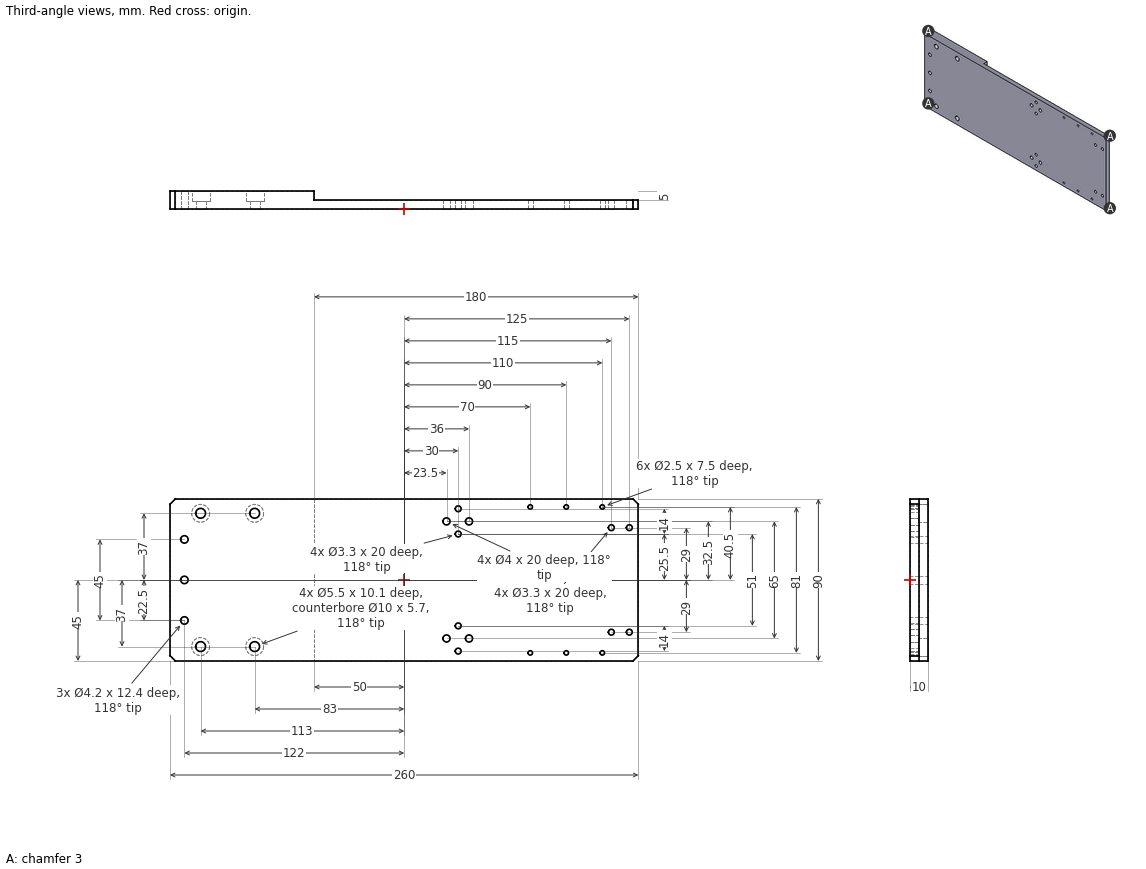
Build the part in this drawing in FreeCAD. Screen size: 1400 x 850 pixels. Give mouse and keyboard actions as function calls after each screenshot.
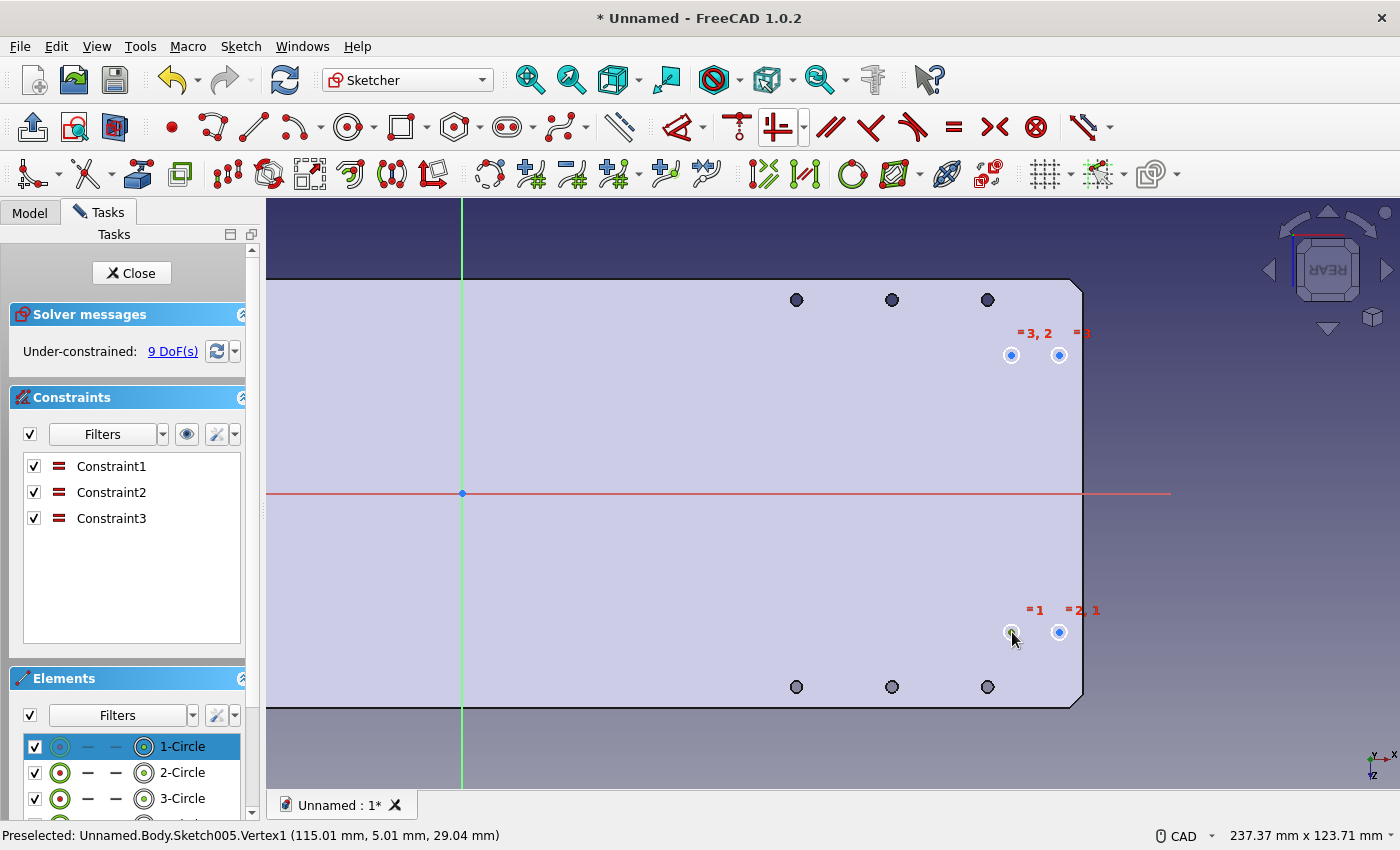
click(1059, 632)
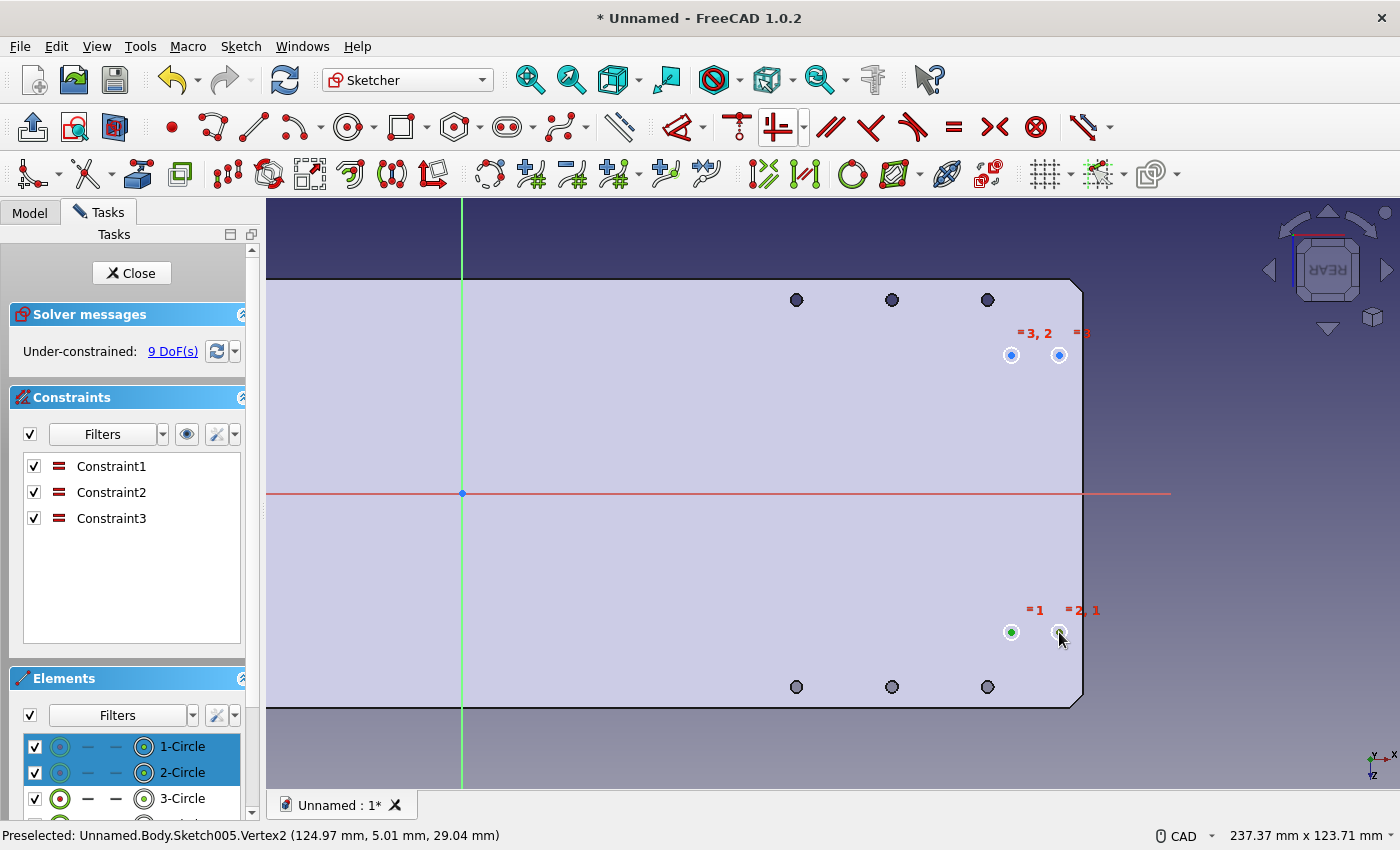
click(804, 128)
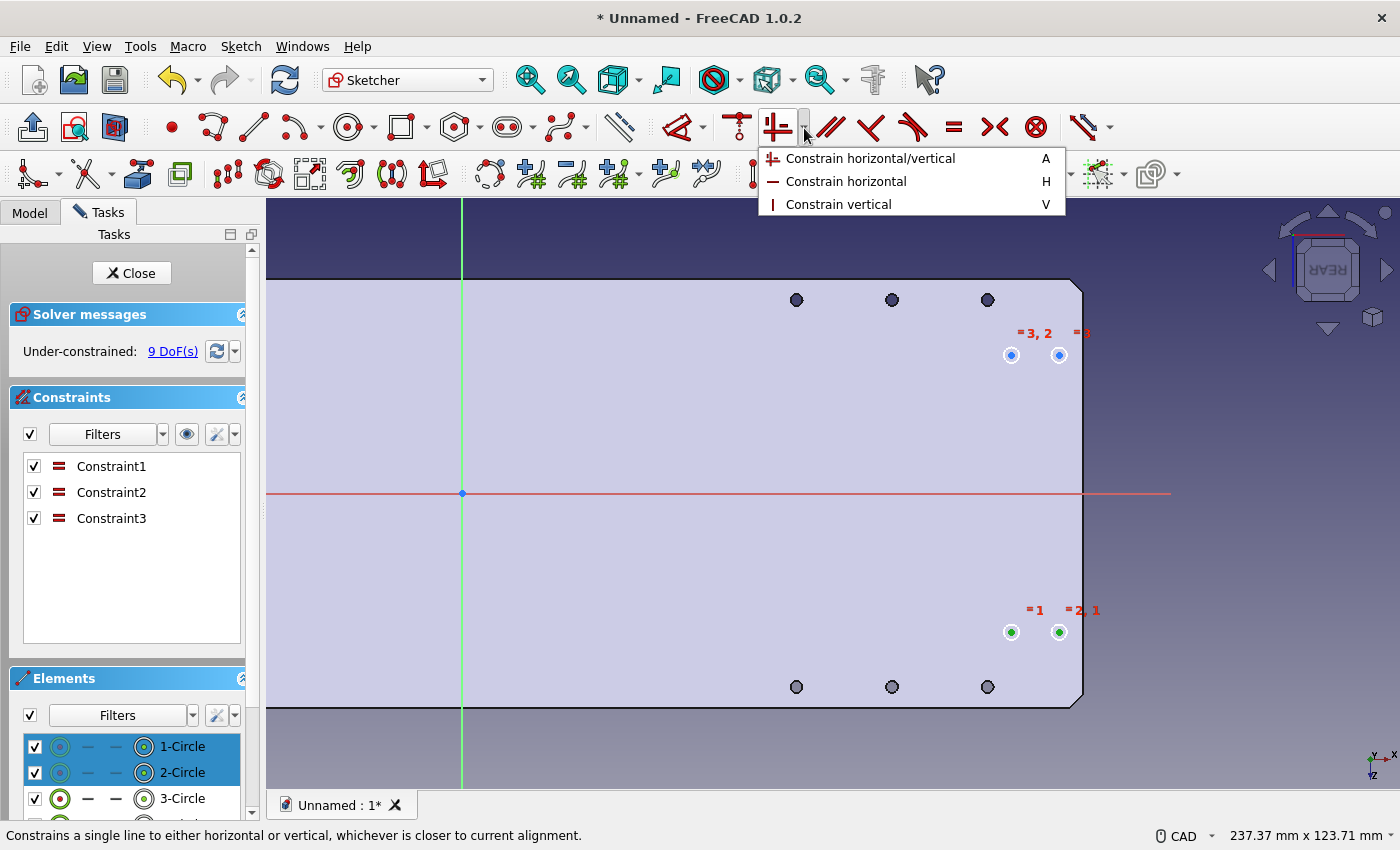
click(912, 182)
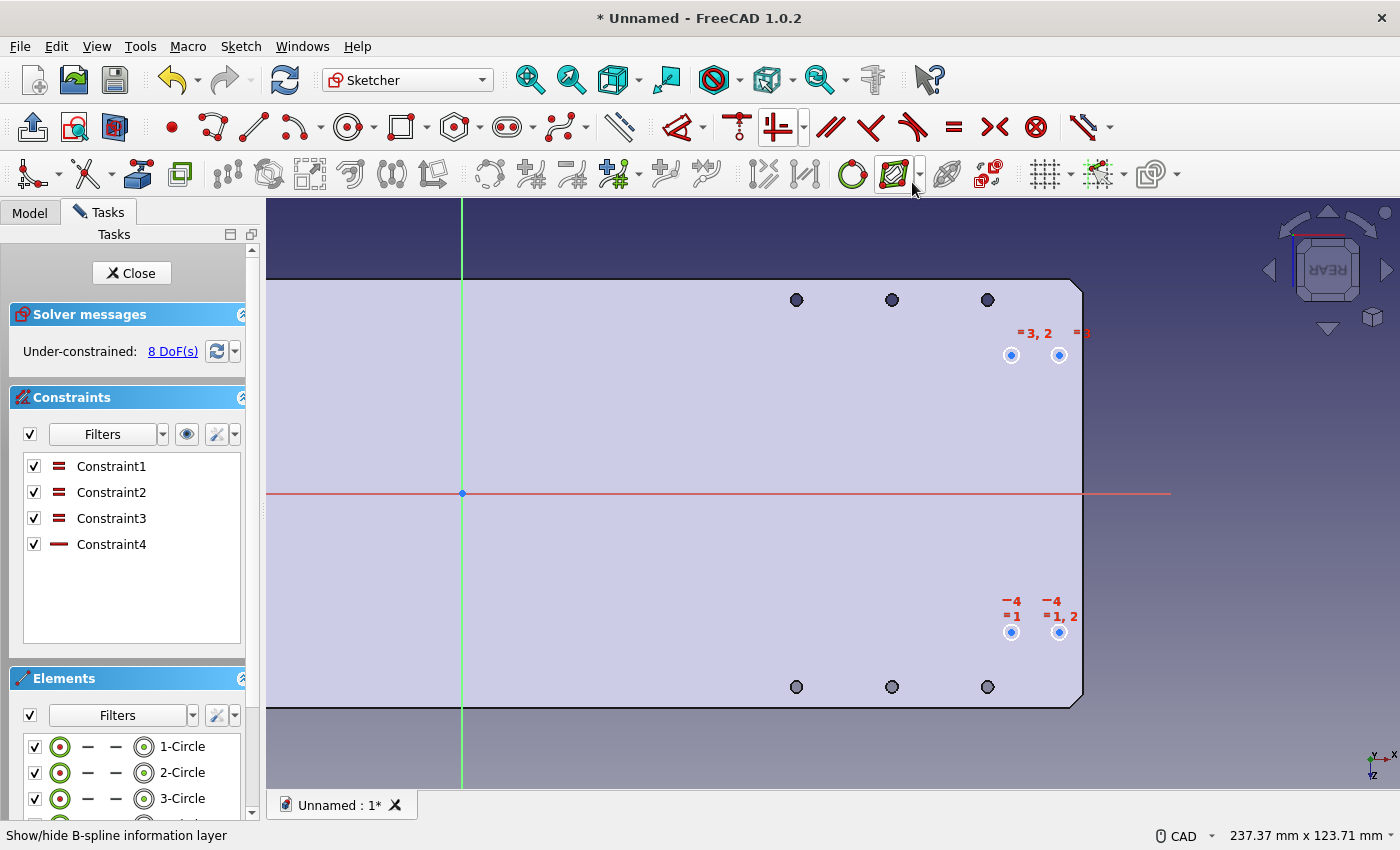
click(1012, 632)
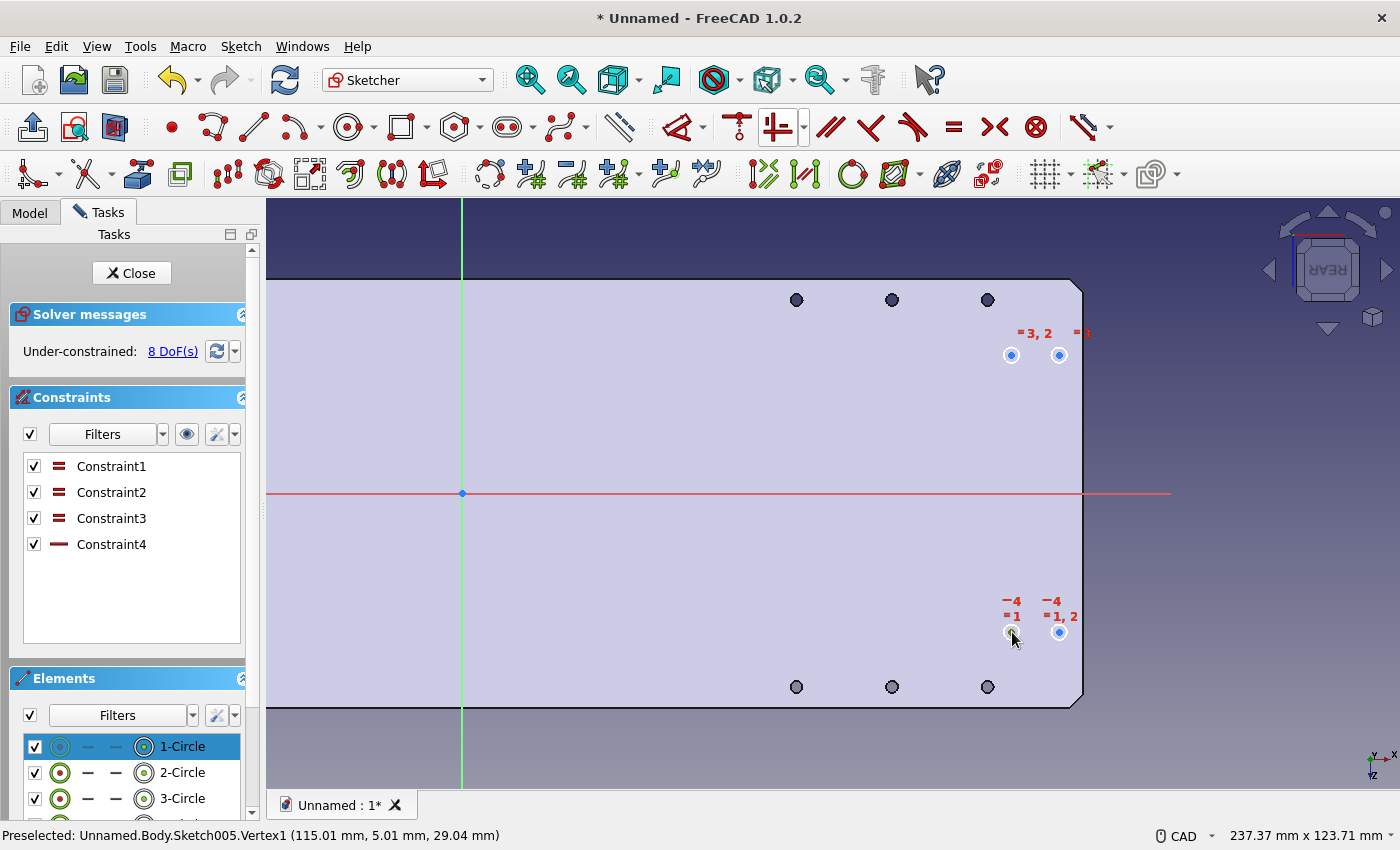
click(1012, 355)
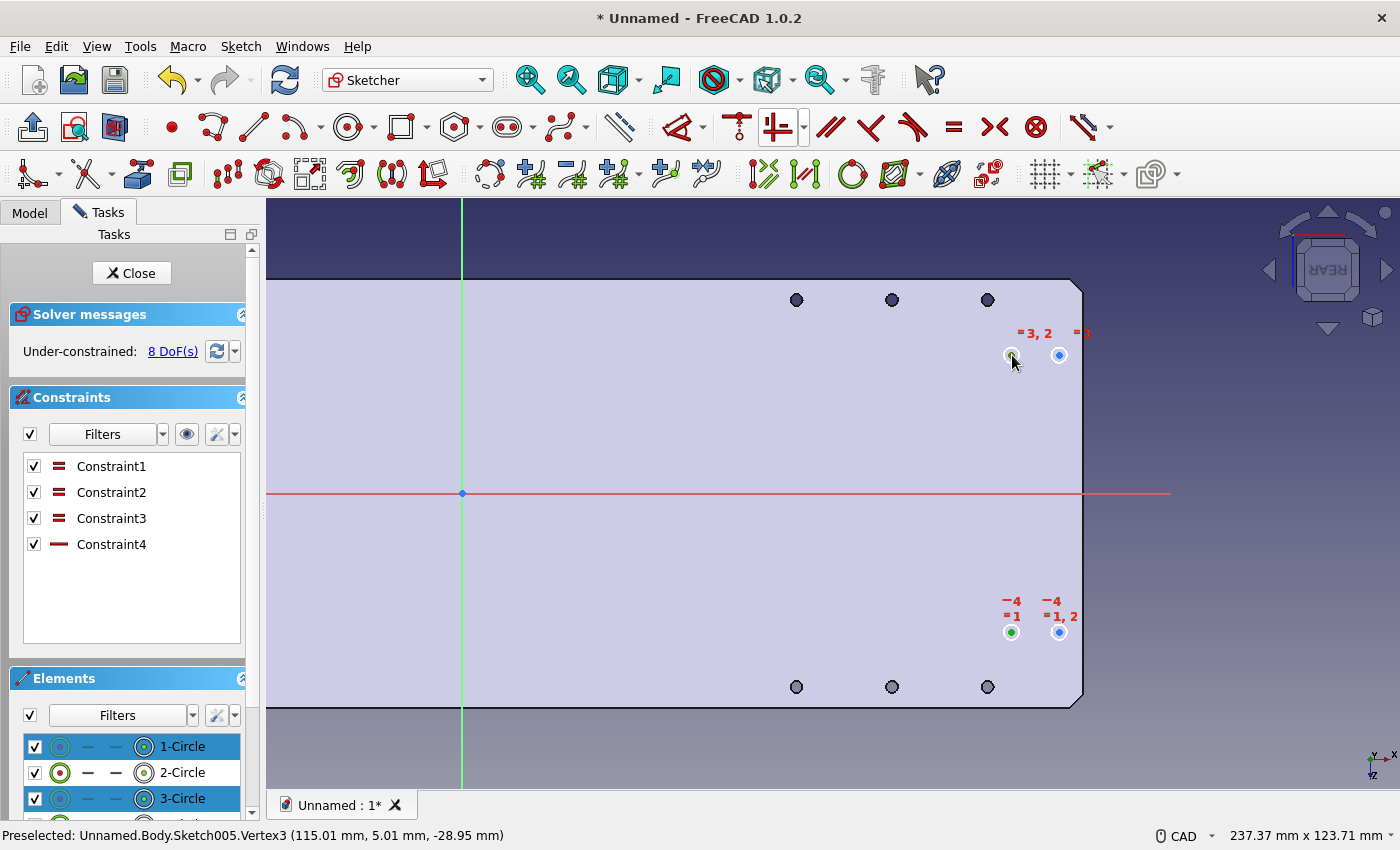
key(v)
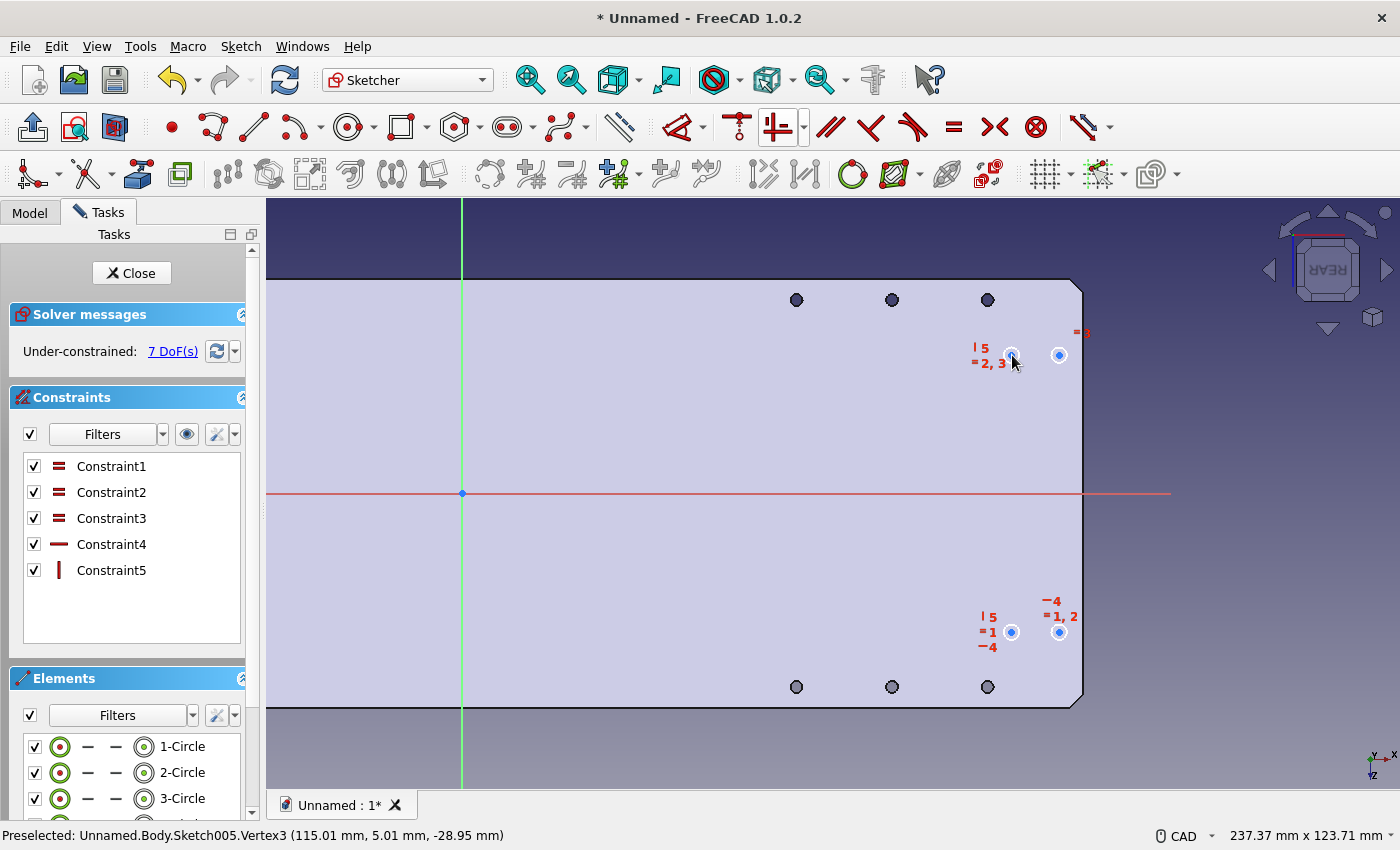
click(1059, 632)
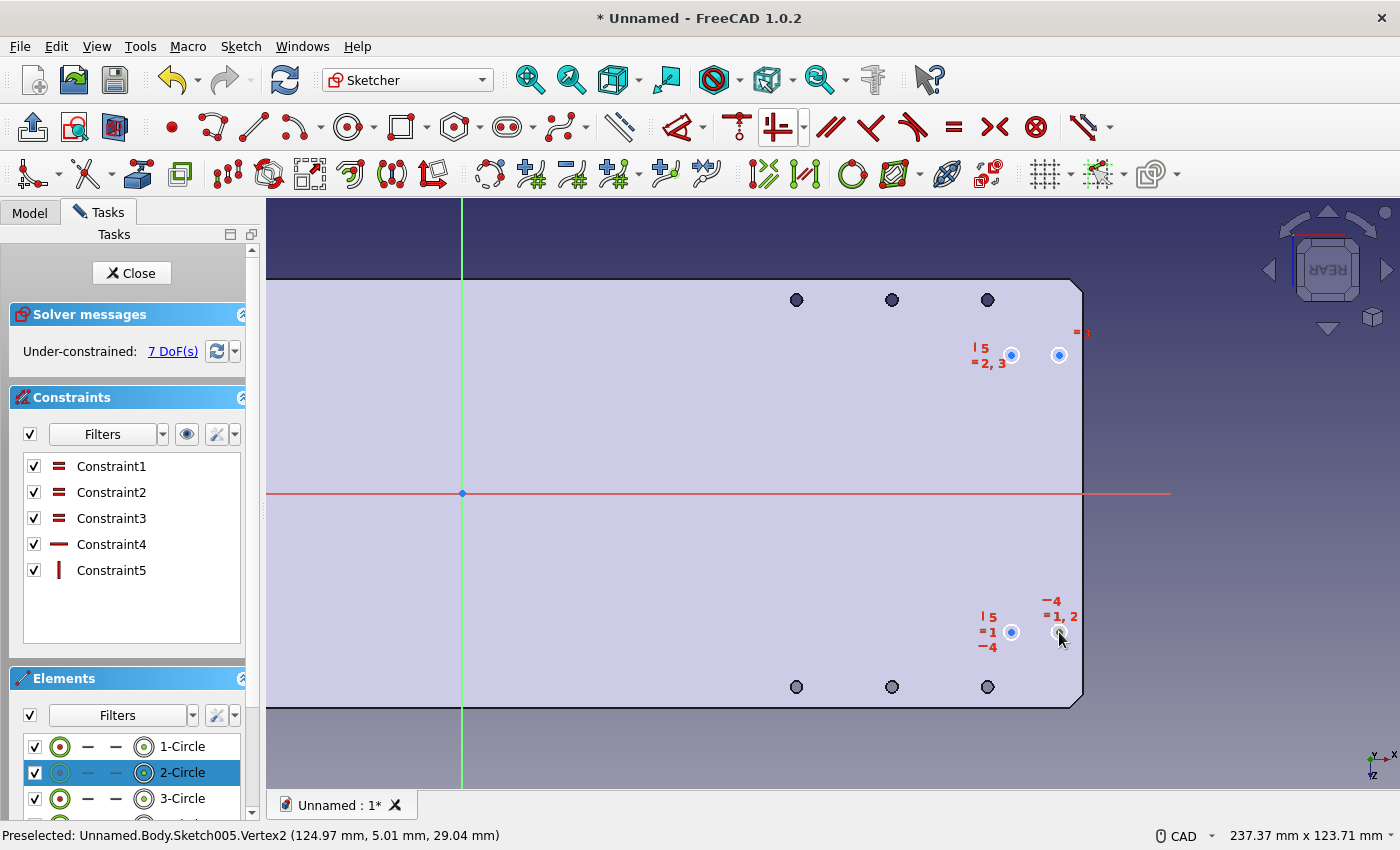
click(1059, 355)